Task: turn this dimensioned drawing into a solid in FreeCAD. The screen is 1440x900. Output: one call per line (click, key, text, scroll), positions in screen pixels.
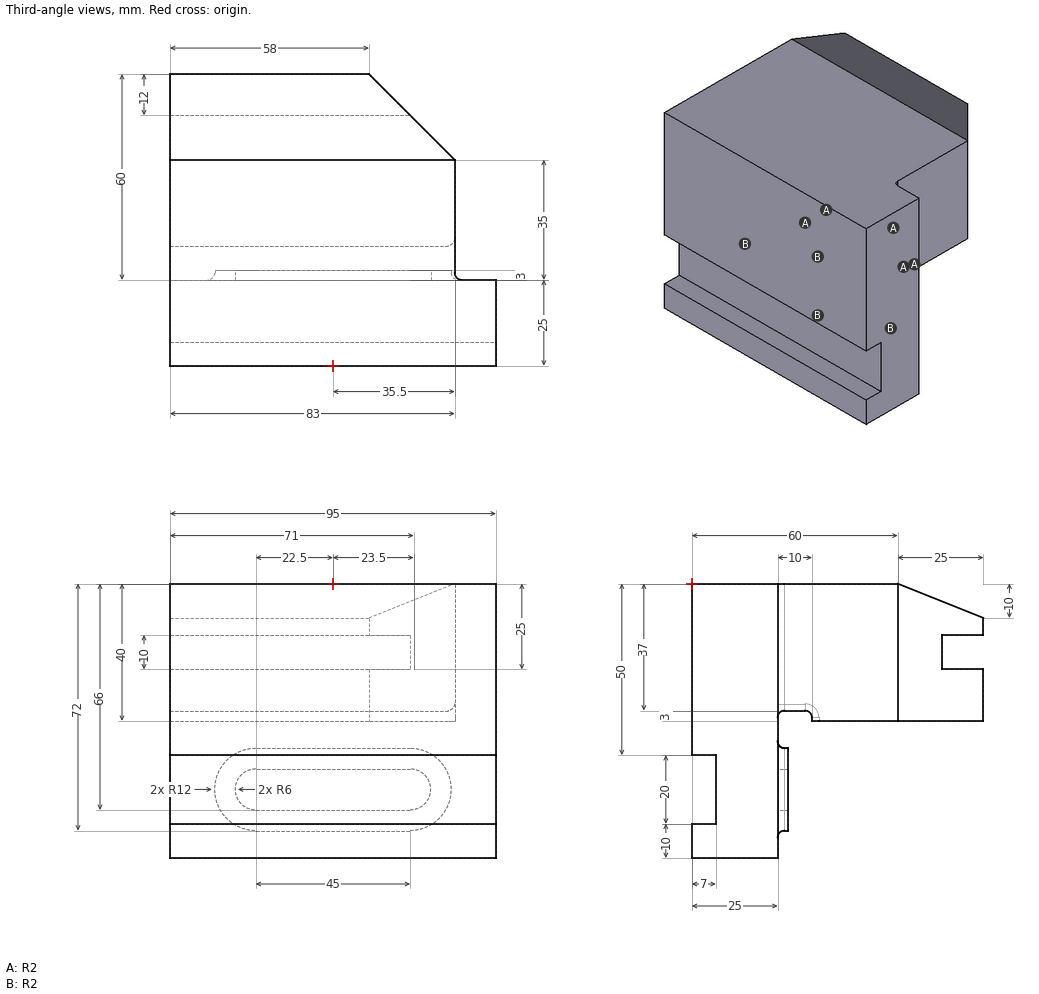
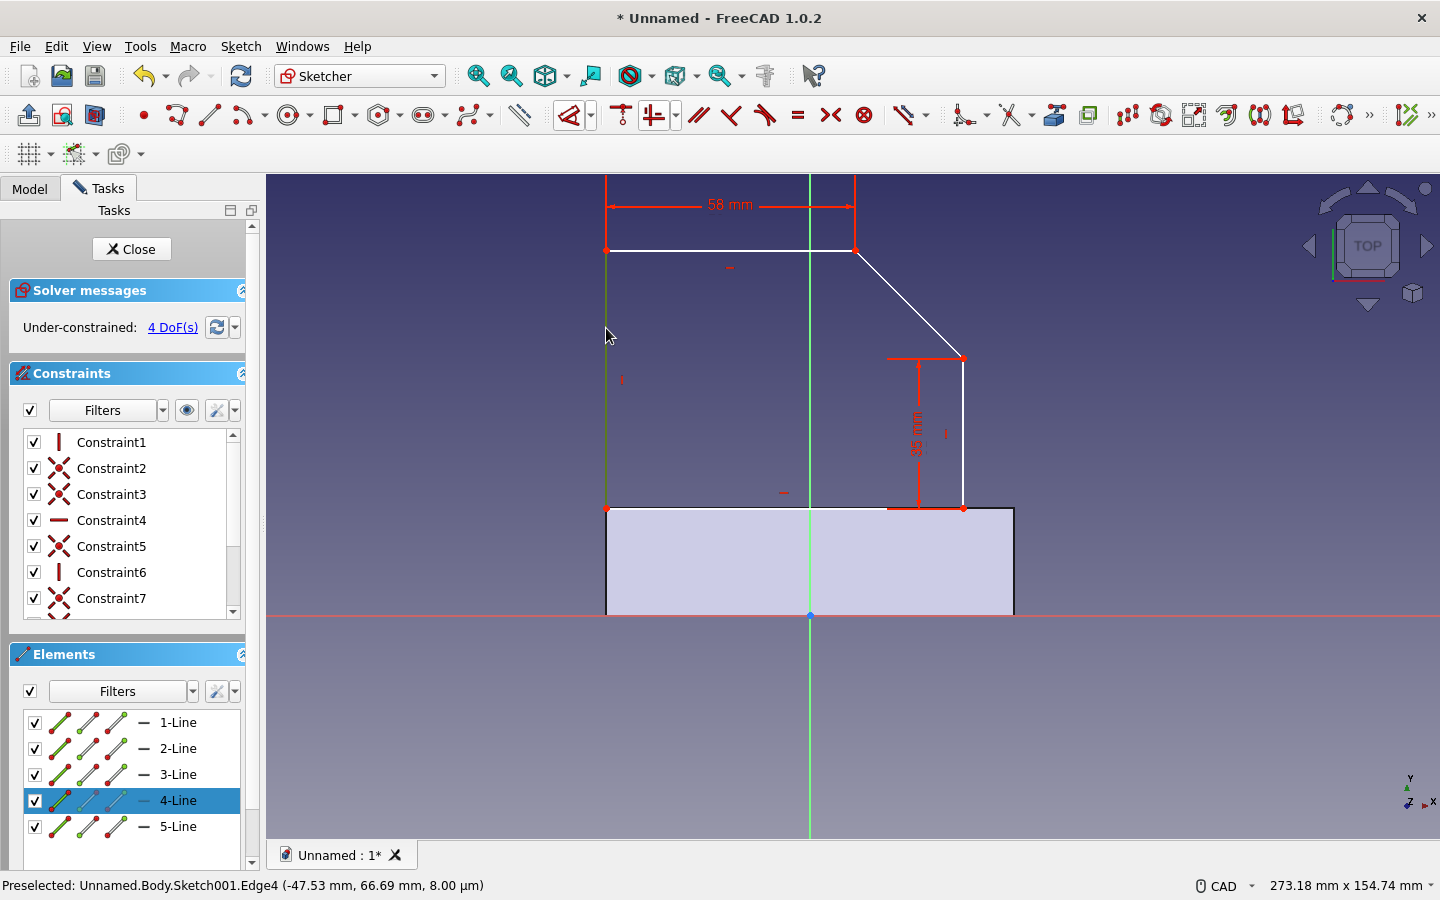
click(590, 116)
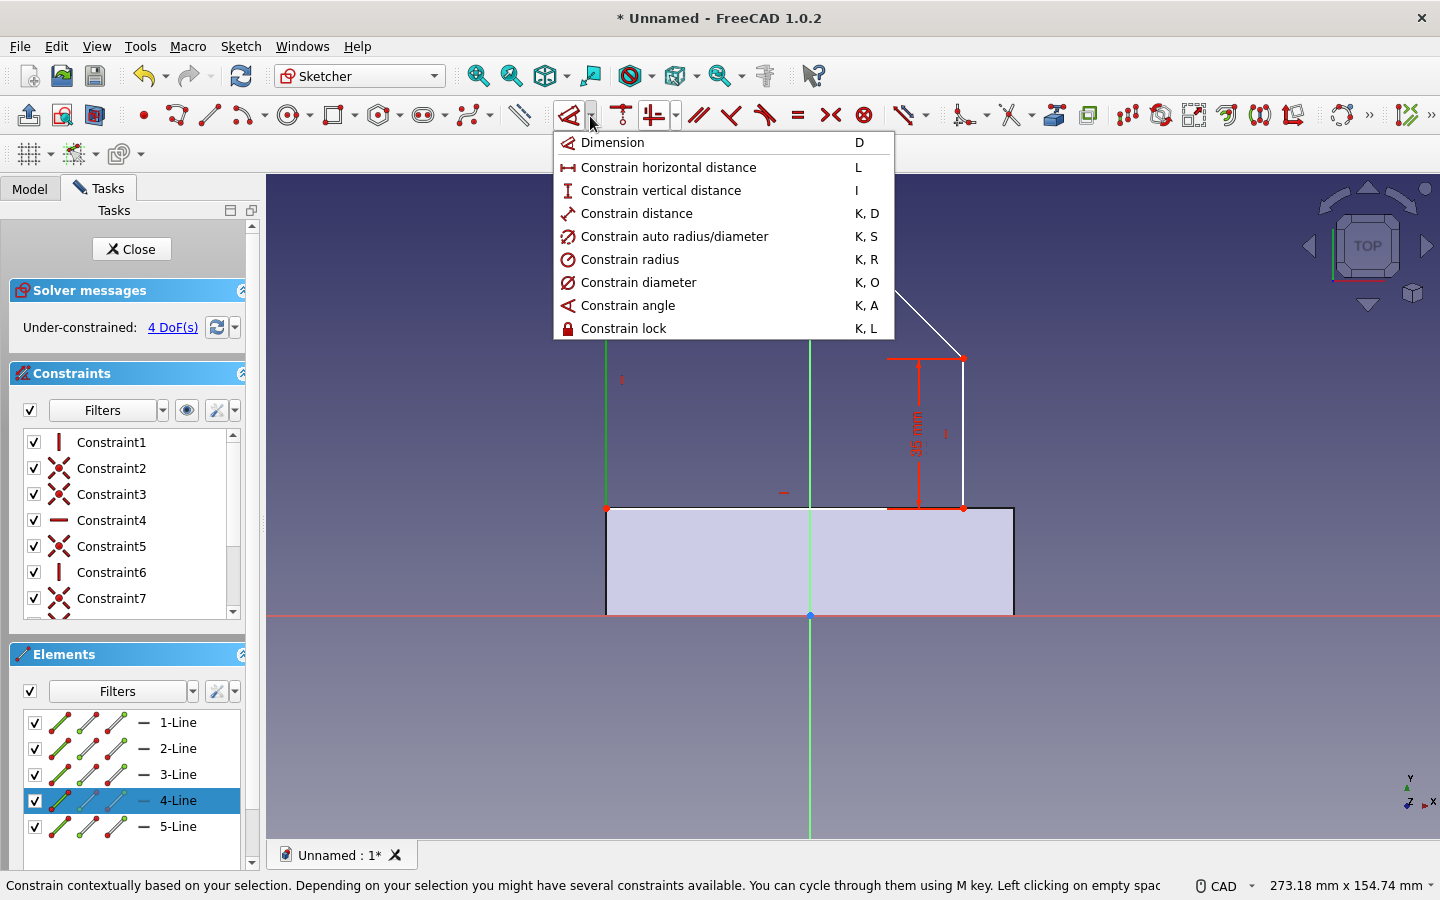
click(724, 190)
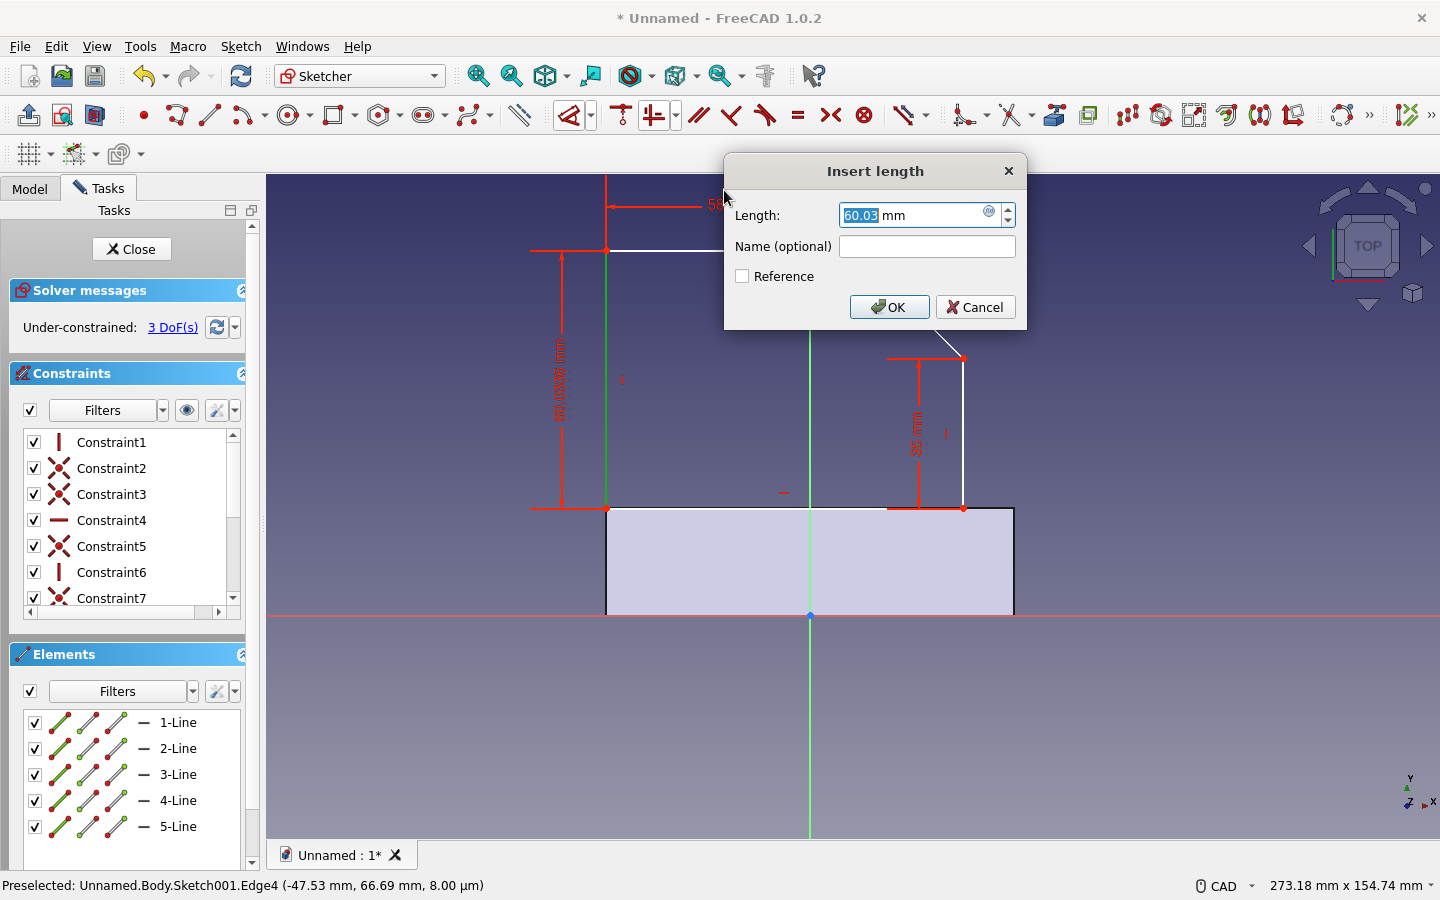
text(60)
key(Return)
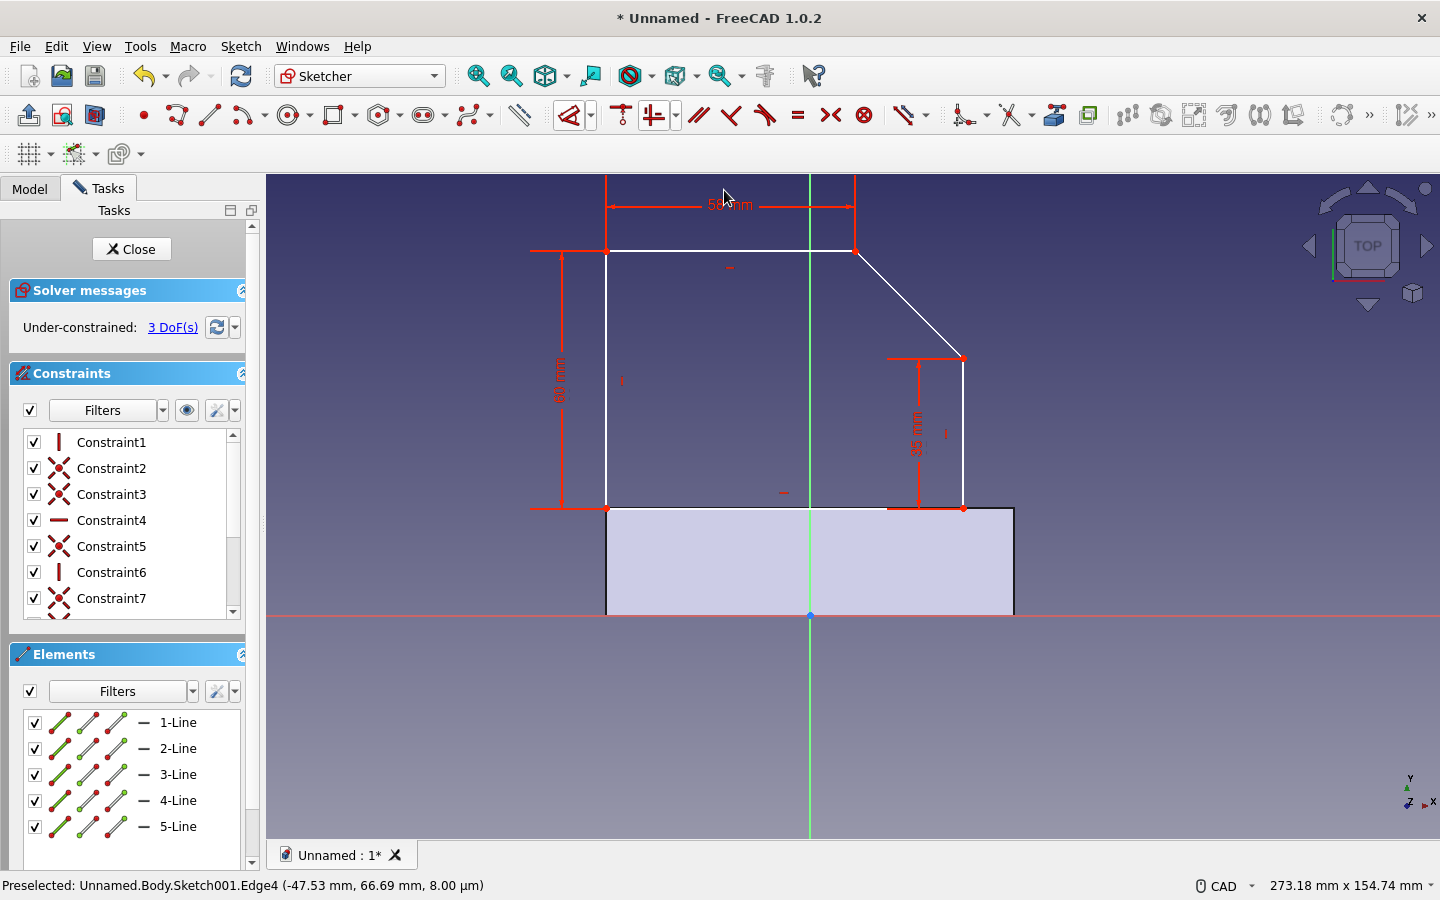
click(713, 509)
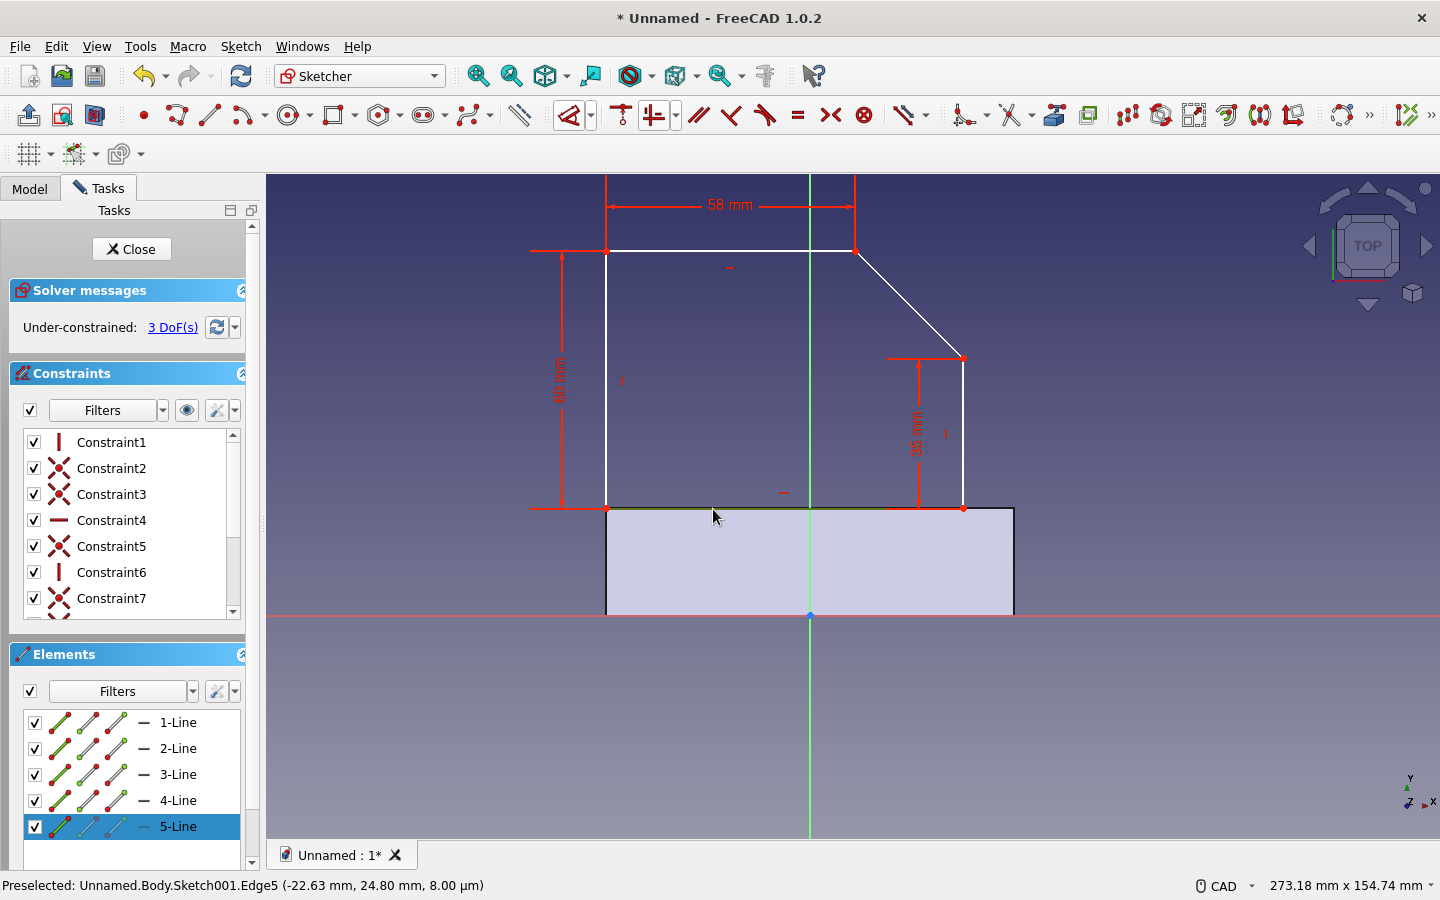
key(l)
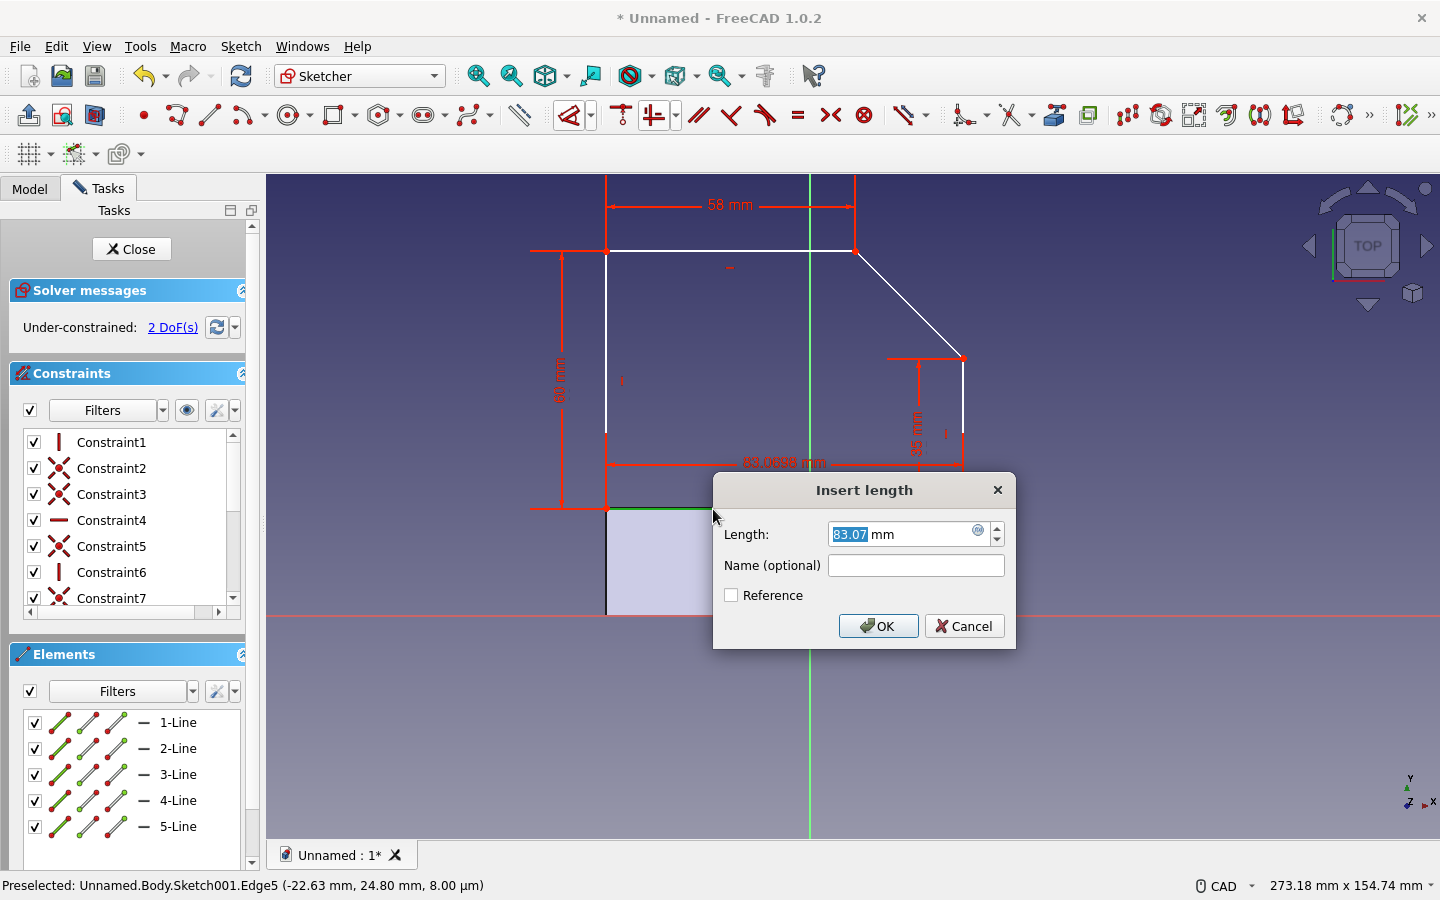
text(83)
key(Return)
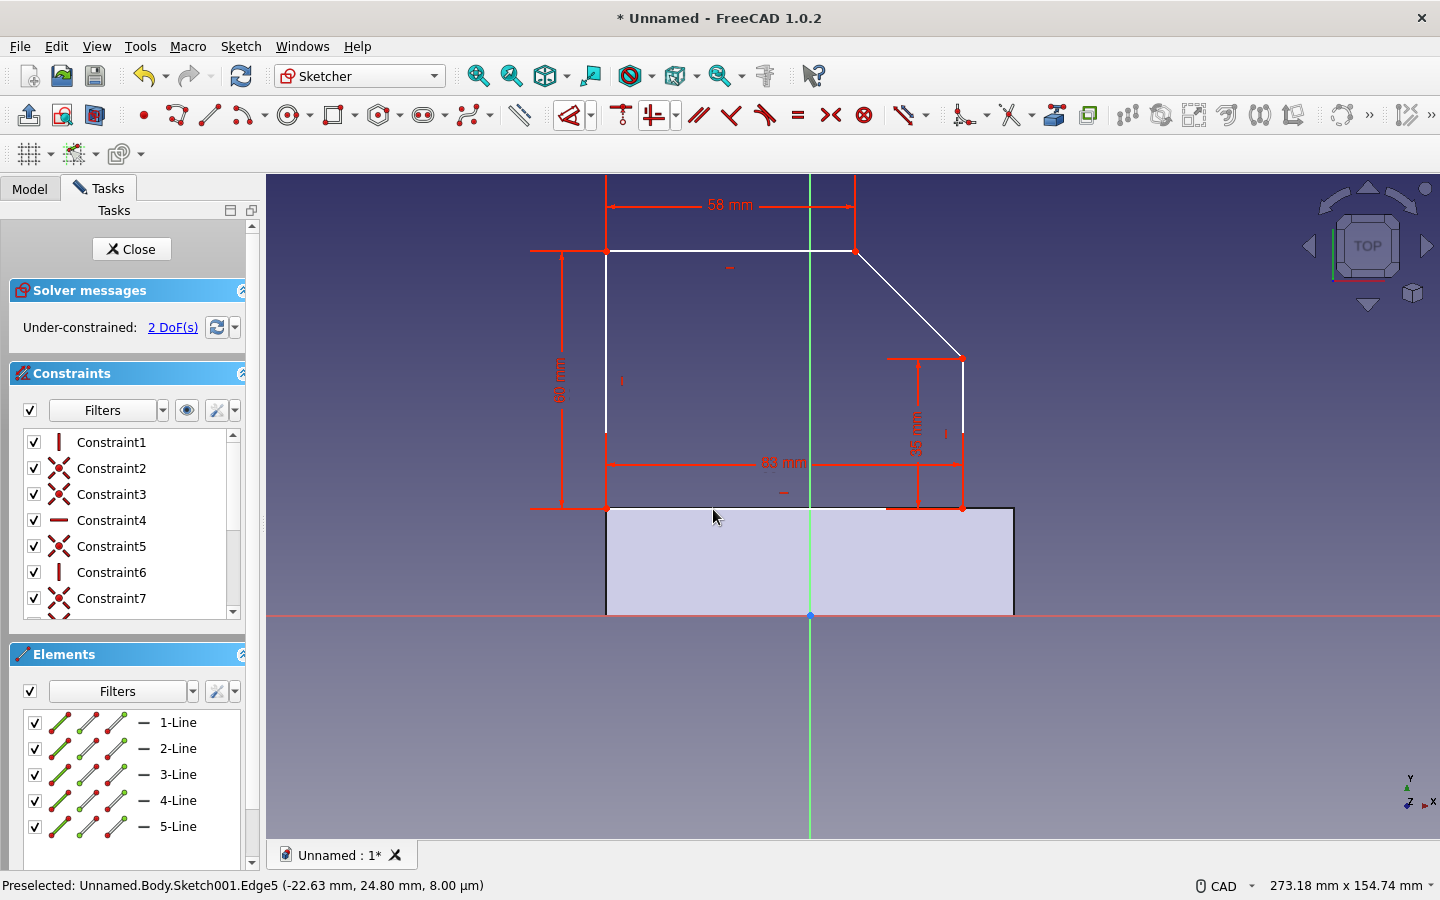
click(963, 509)